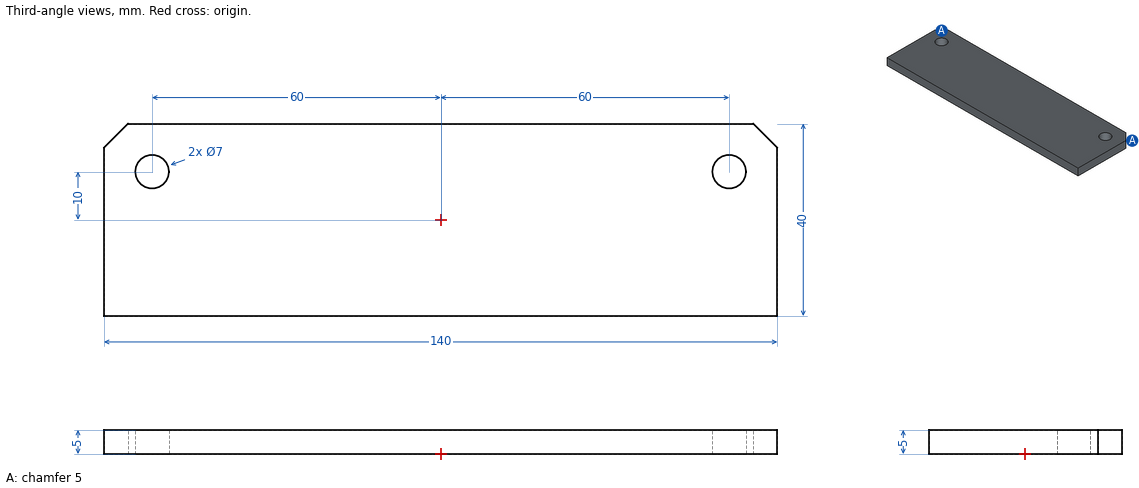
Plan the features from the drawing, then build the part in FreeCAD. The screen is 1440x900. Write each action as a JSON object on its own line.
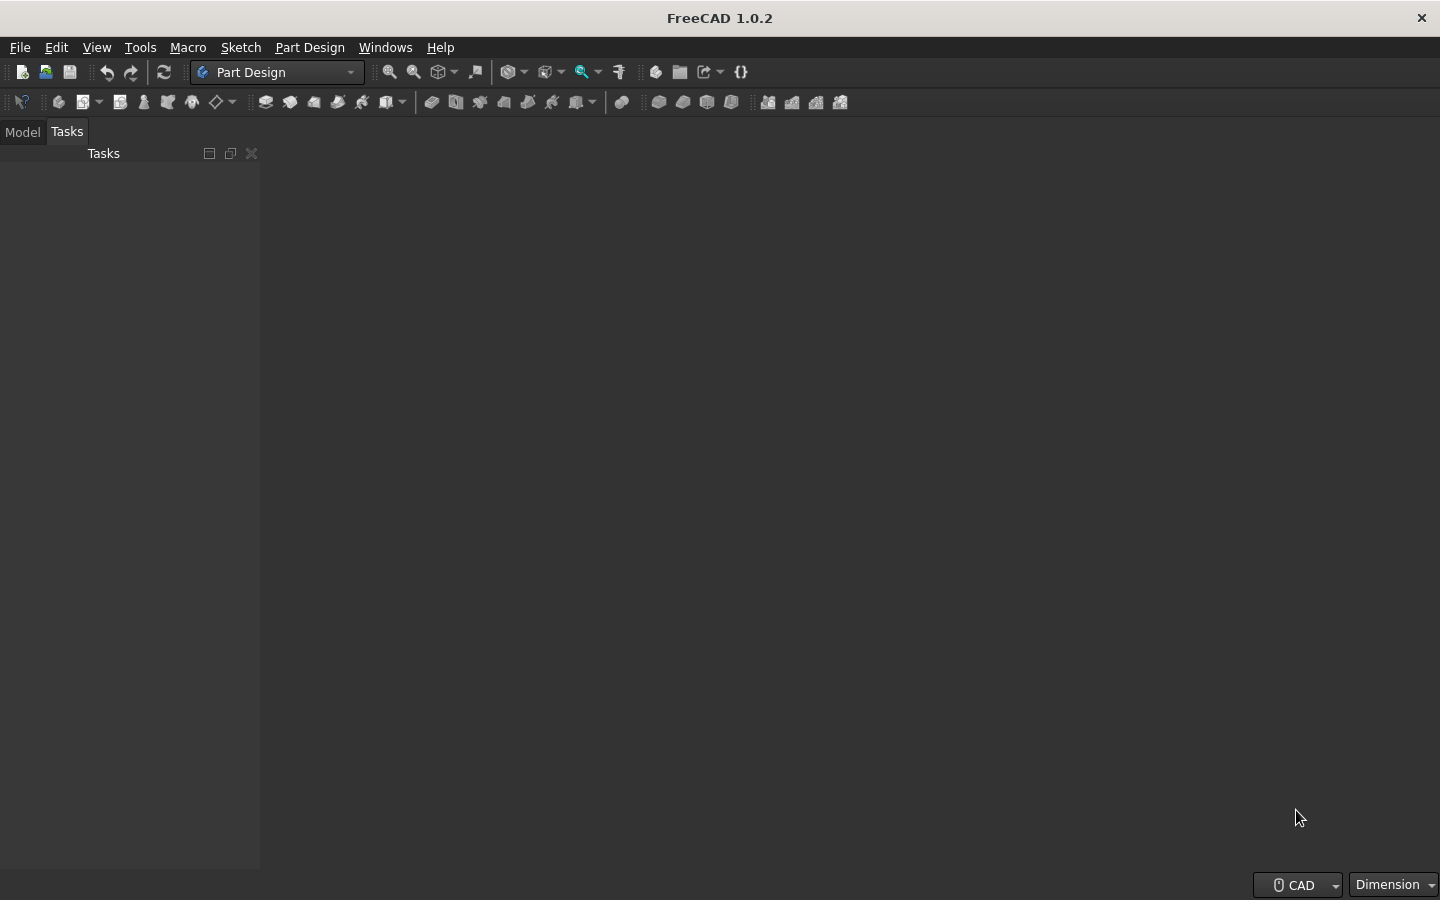
{"action": "left_click", "coordinate": [22, 72]}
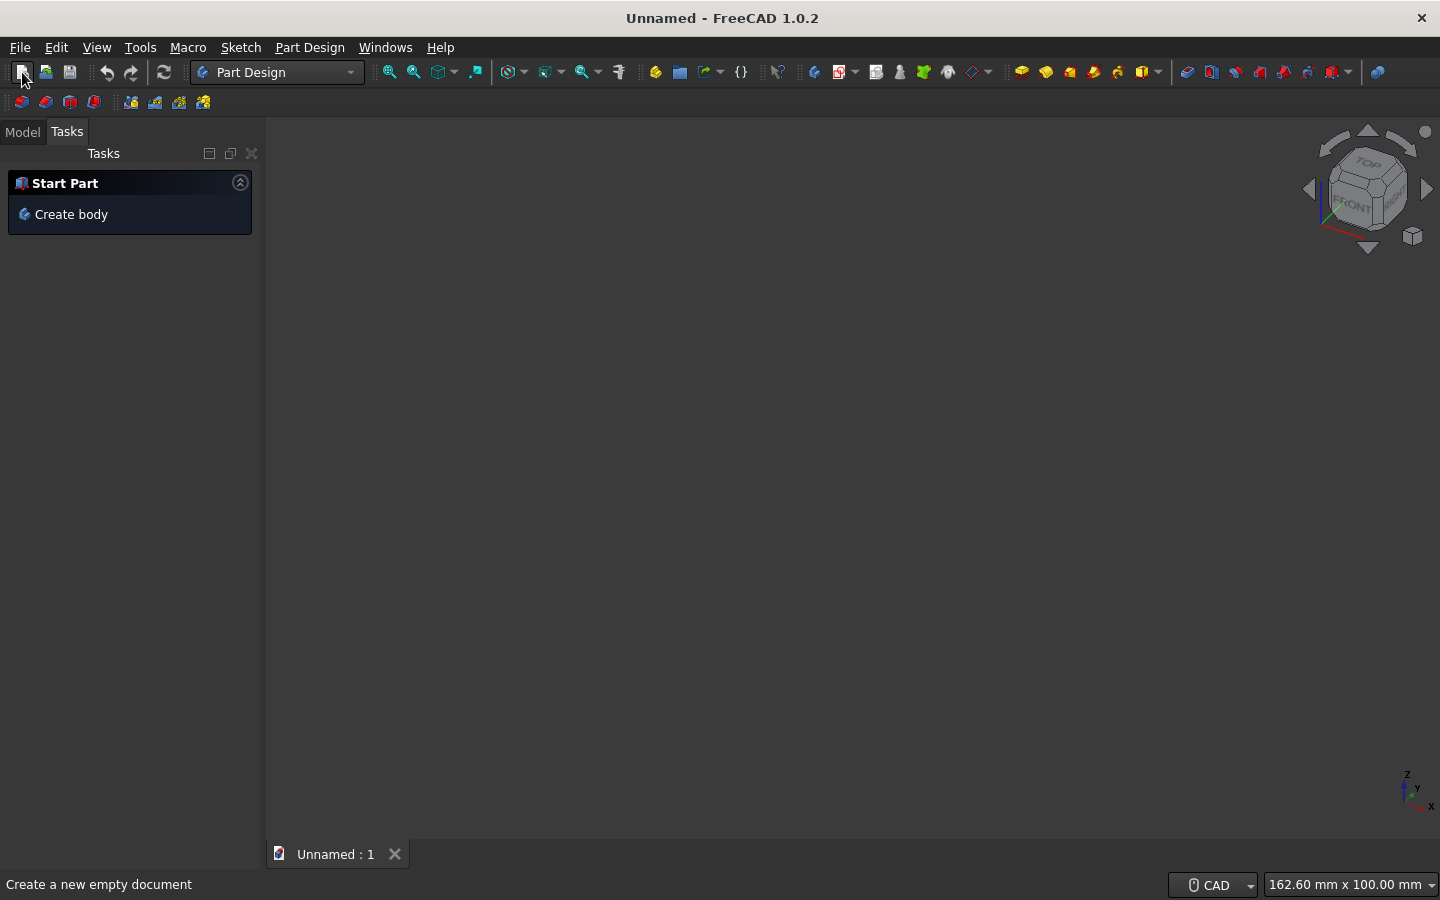
{"action": "left_click", "coordinate": [840, 72]}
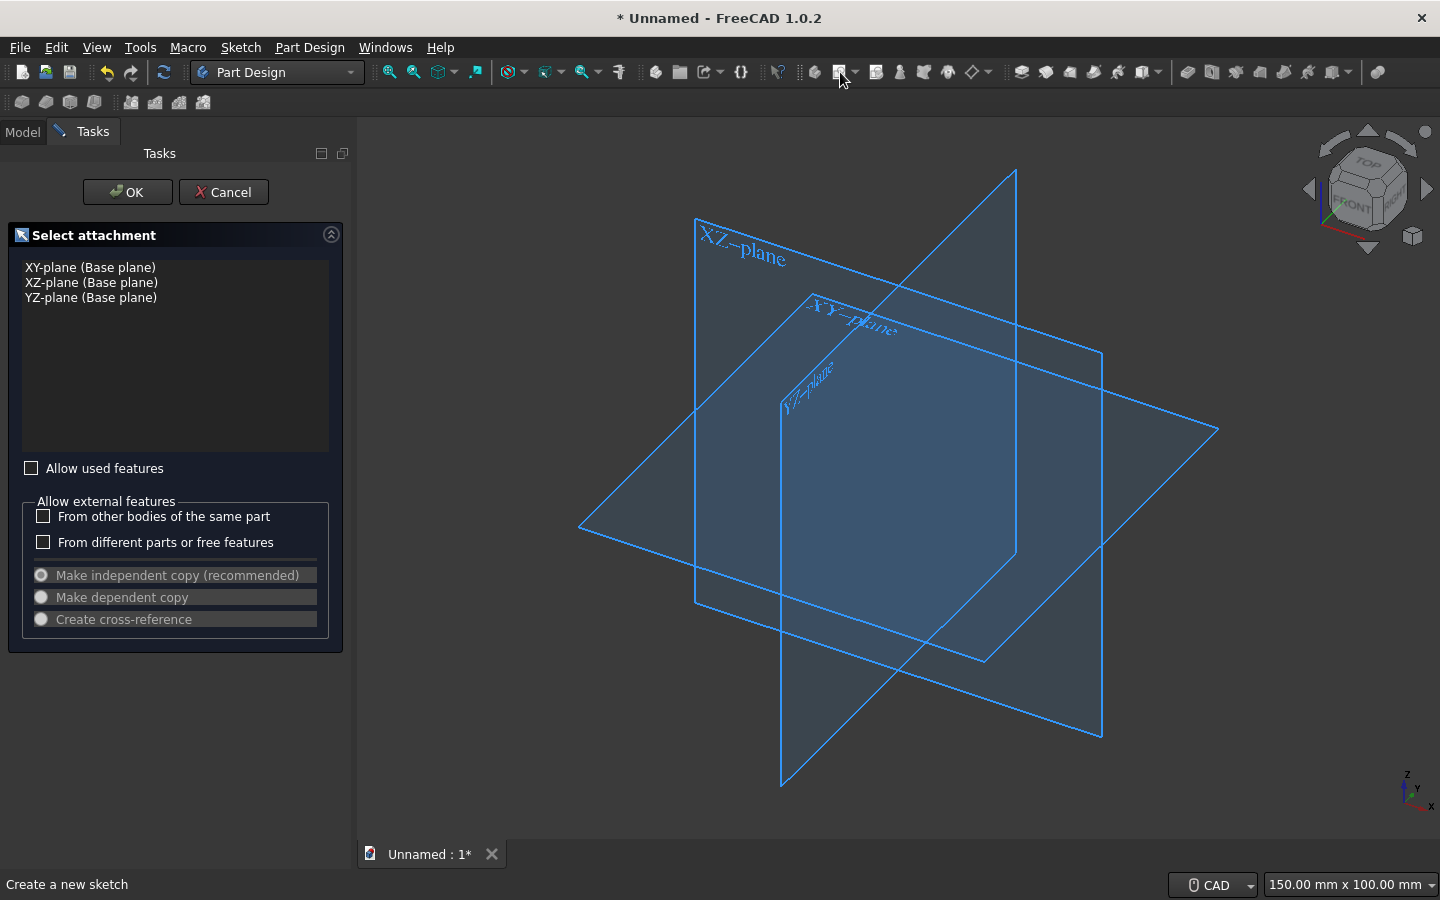
{"action": "left_click", "coordinate": [82, 268]}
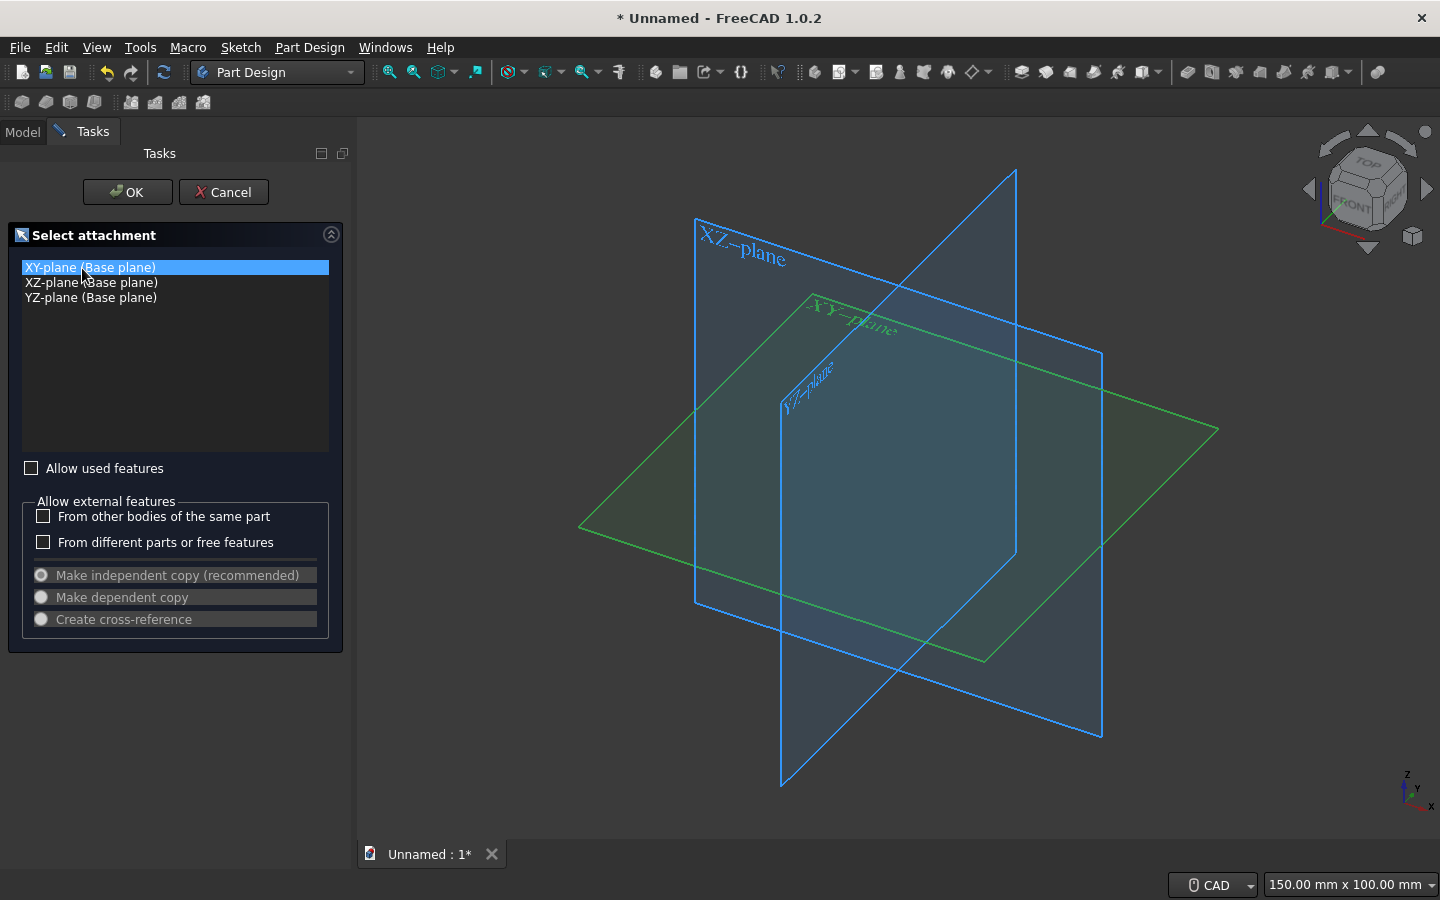
{"action": "left_click", "coordinate": [128, 192]}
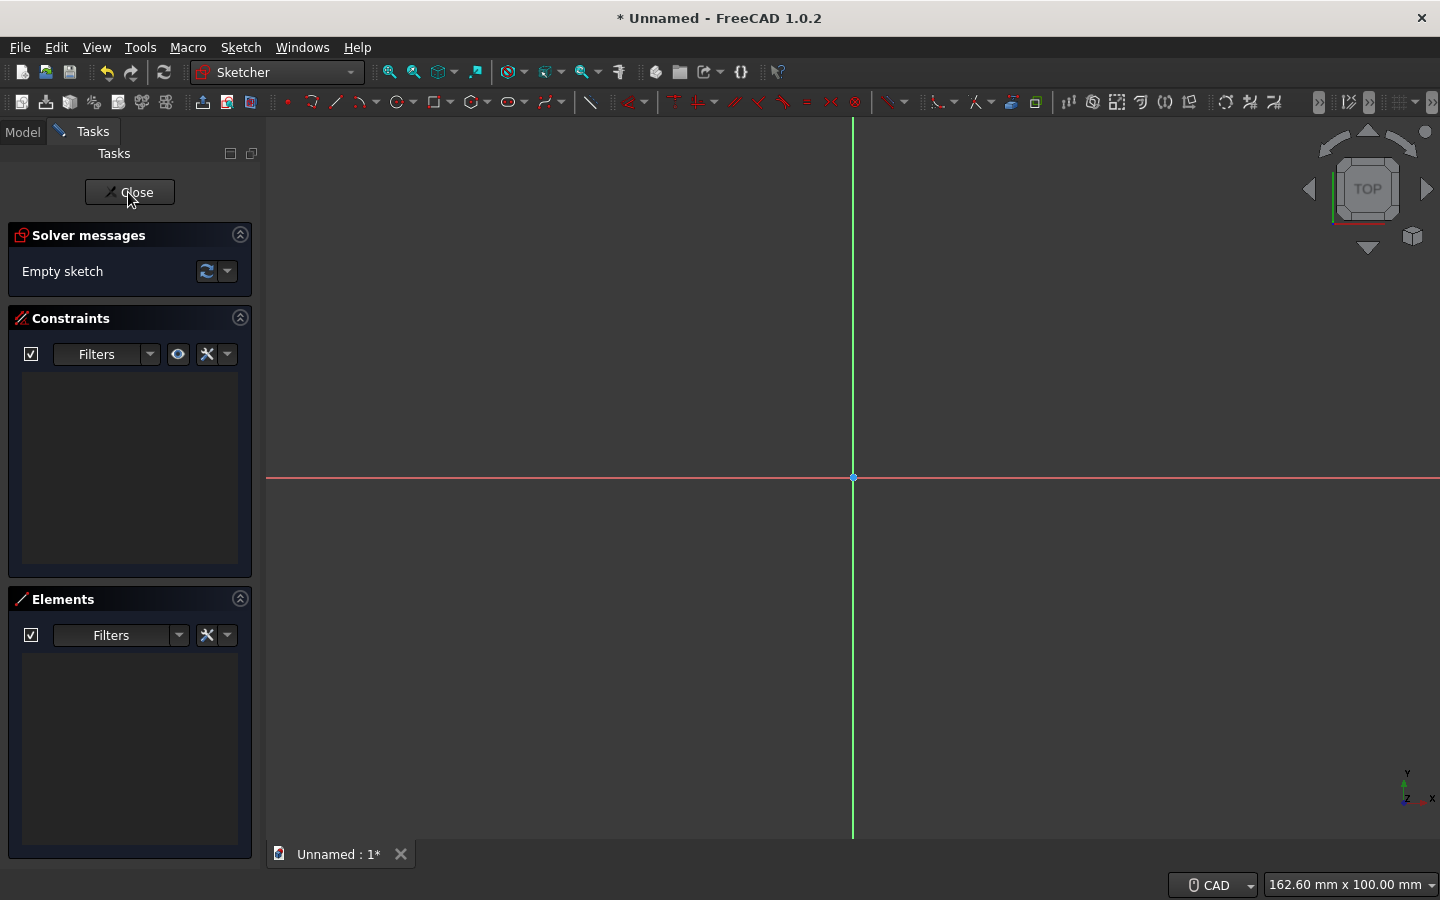
{"action": "scroll", "coordinate": [645, 478], "scroll_direction": "down", "scroll_amount": 2}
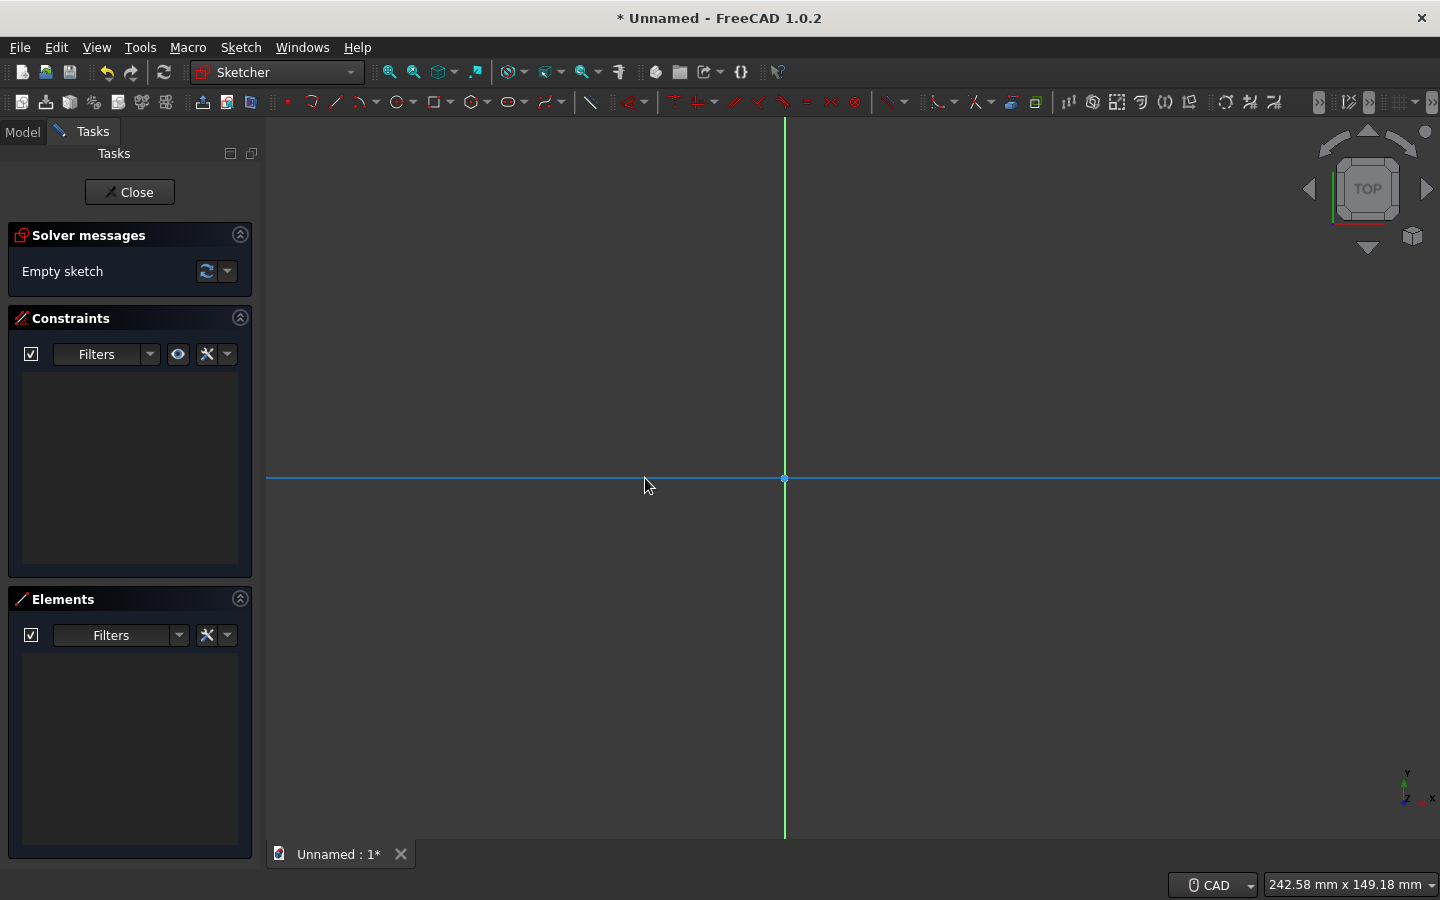
{"action": "key", "text": "g v"}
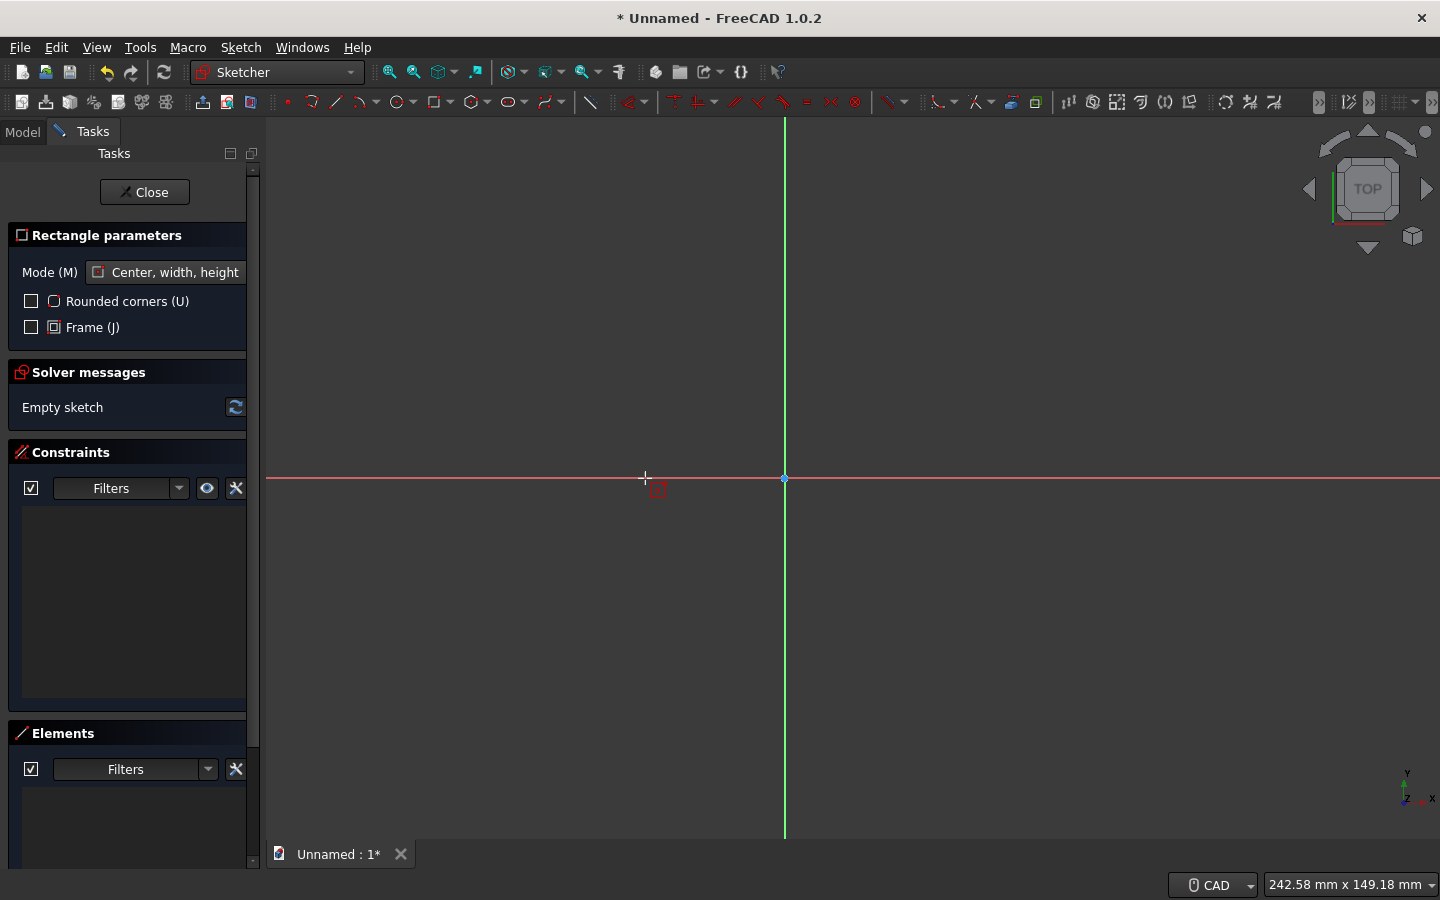
{"action": "left_click", "coordinate": [785, 478]}
{"action": "mouse_move", "coordinate": [1123, 381]}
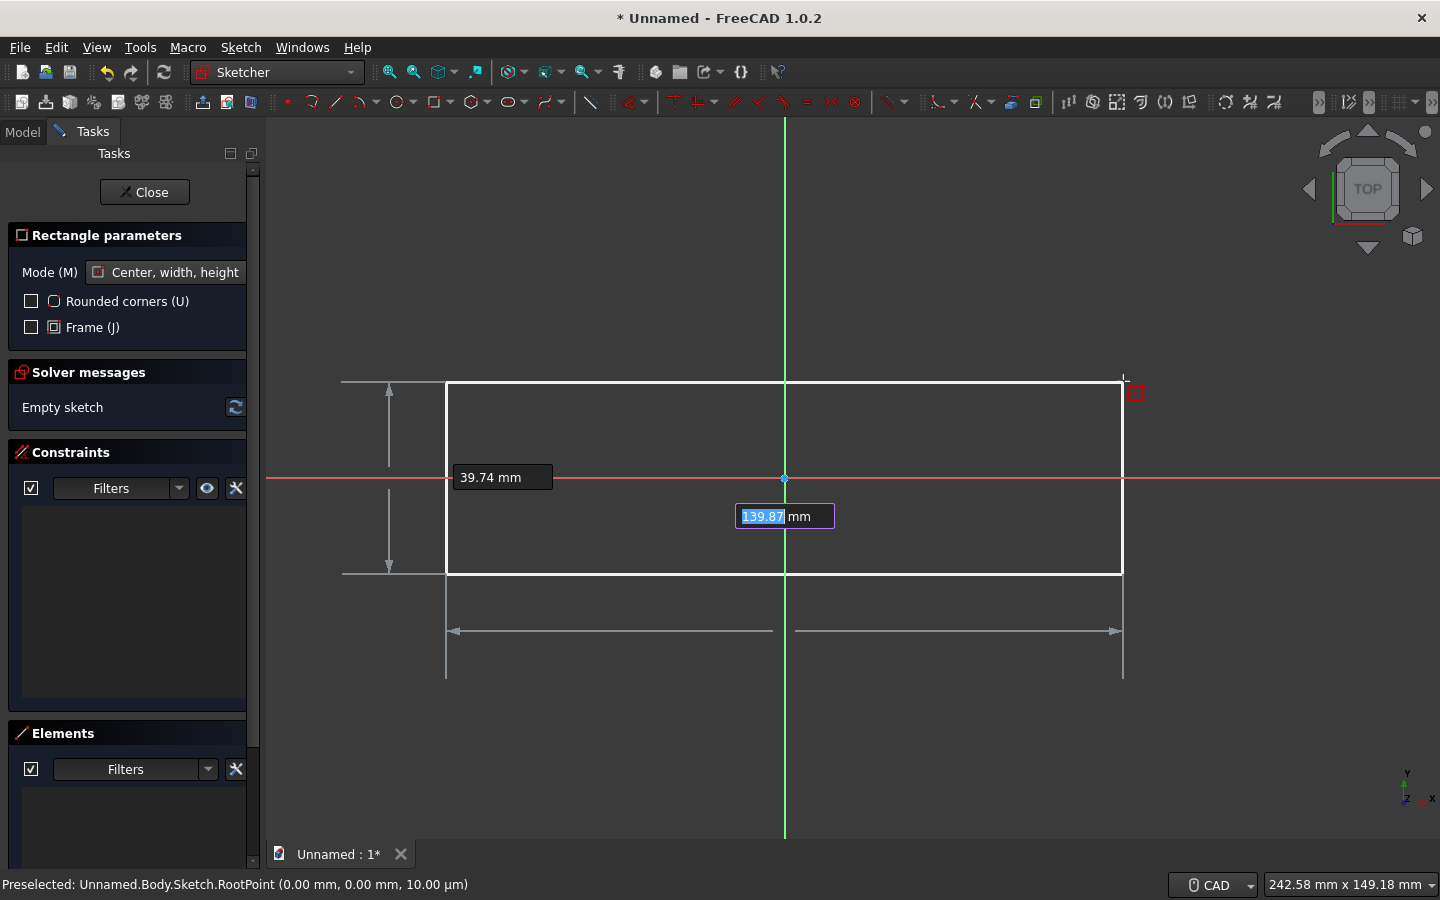
{"action": "type", "text": "140"}
{"action": "key", "text": "Tab"}
{"action": "type", "text": "40"}
{"action": "key", "text": "Return"}
{"action": "key", "text": "Escape"}